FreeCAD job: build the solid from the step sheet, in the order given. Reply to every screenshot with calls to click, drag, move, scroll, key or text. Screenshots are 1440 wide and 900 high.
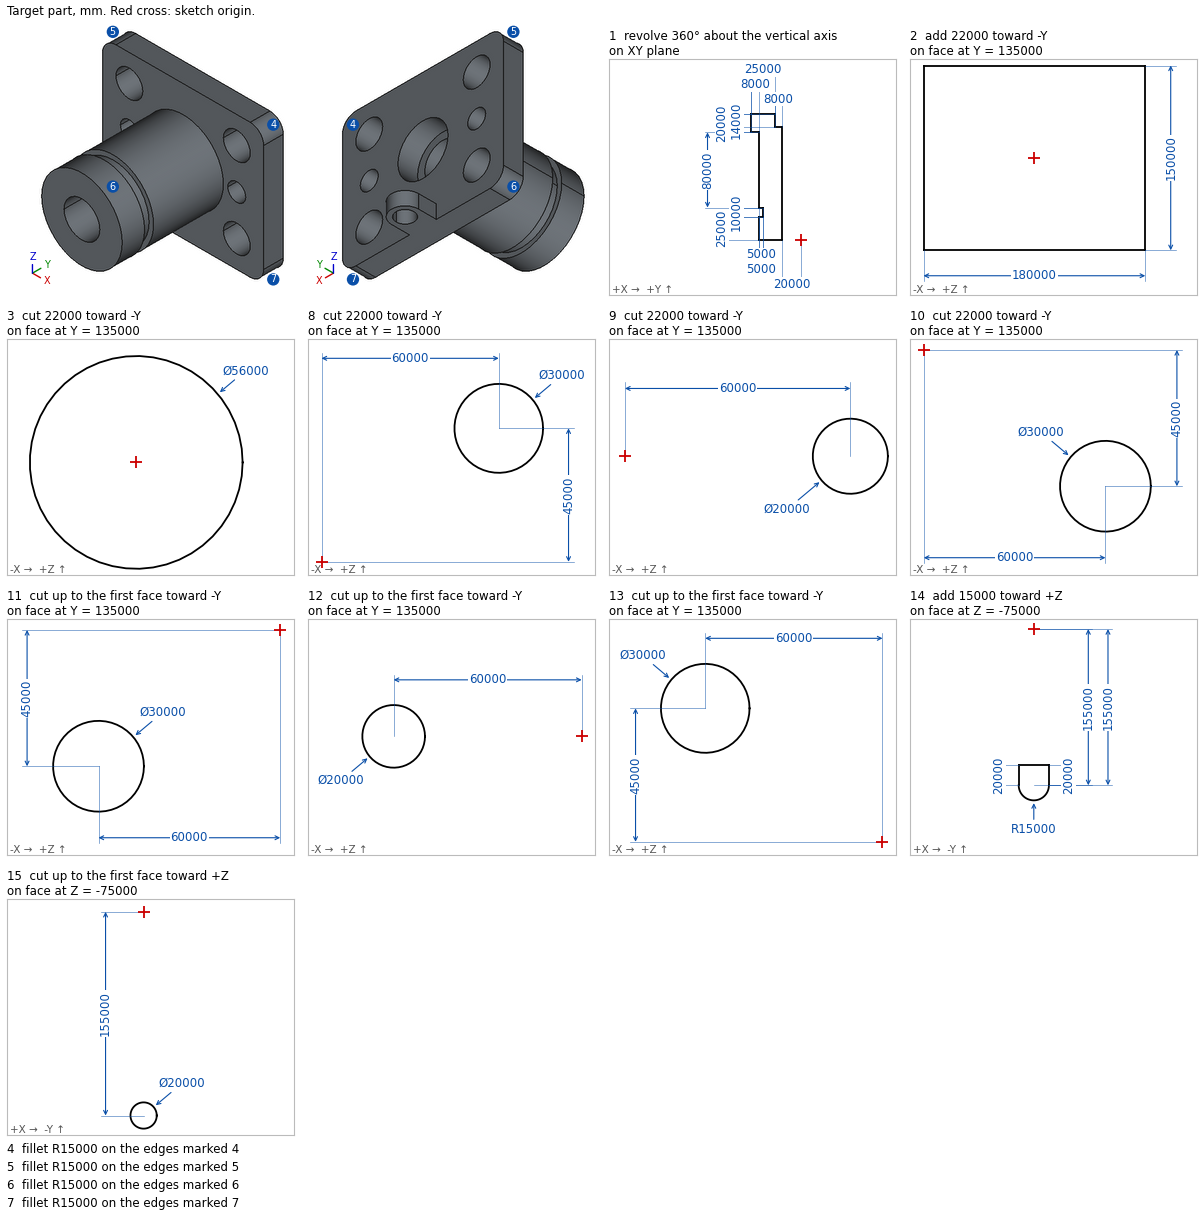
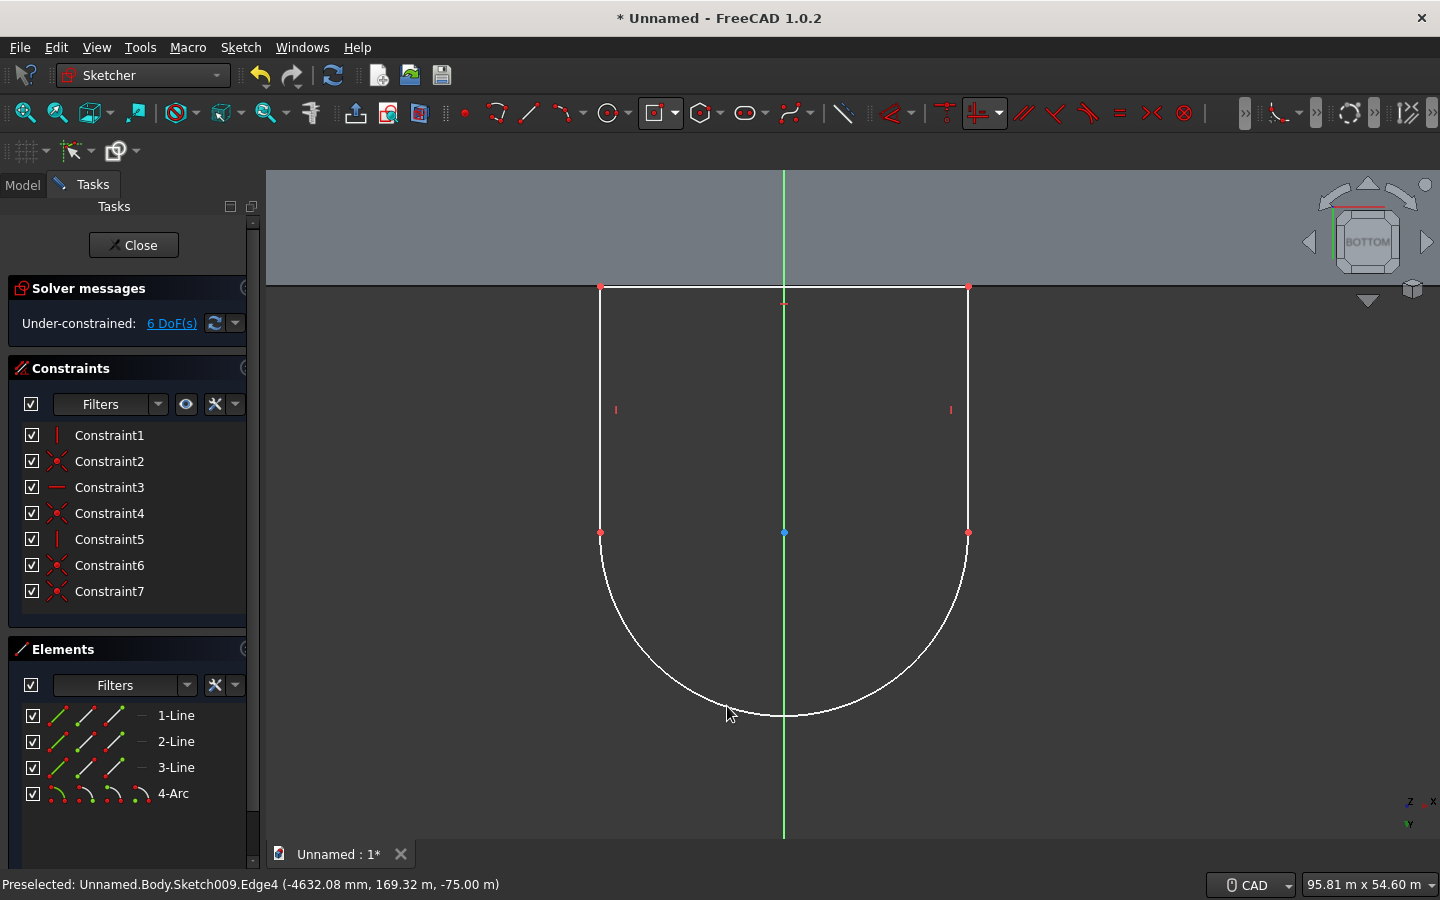
click(784, 532)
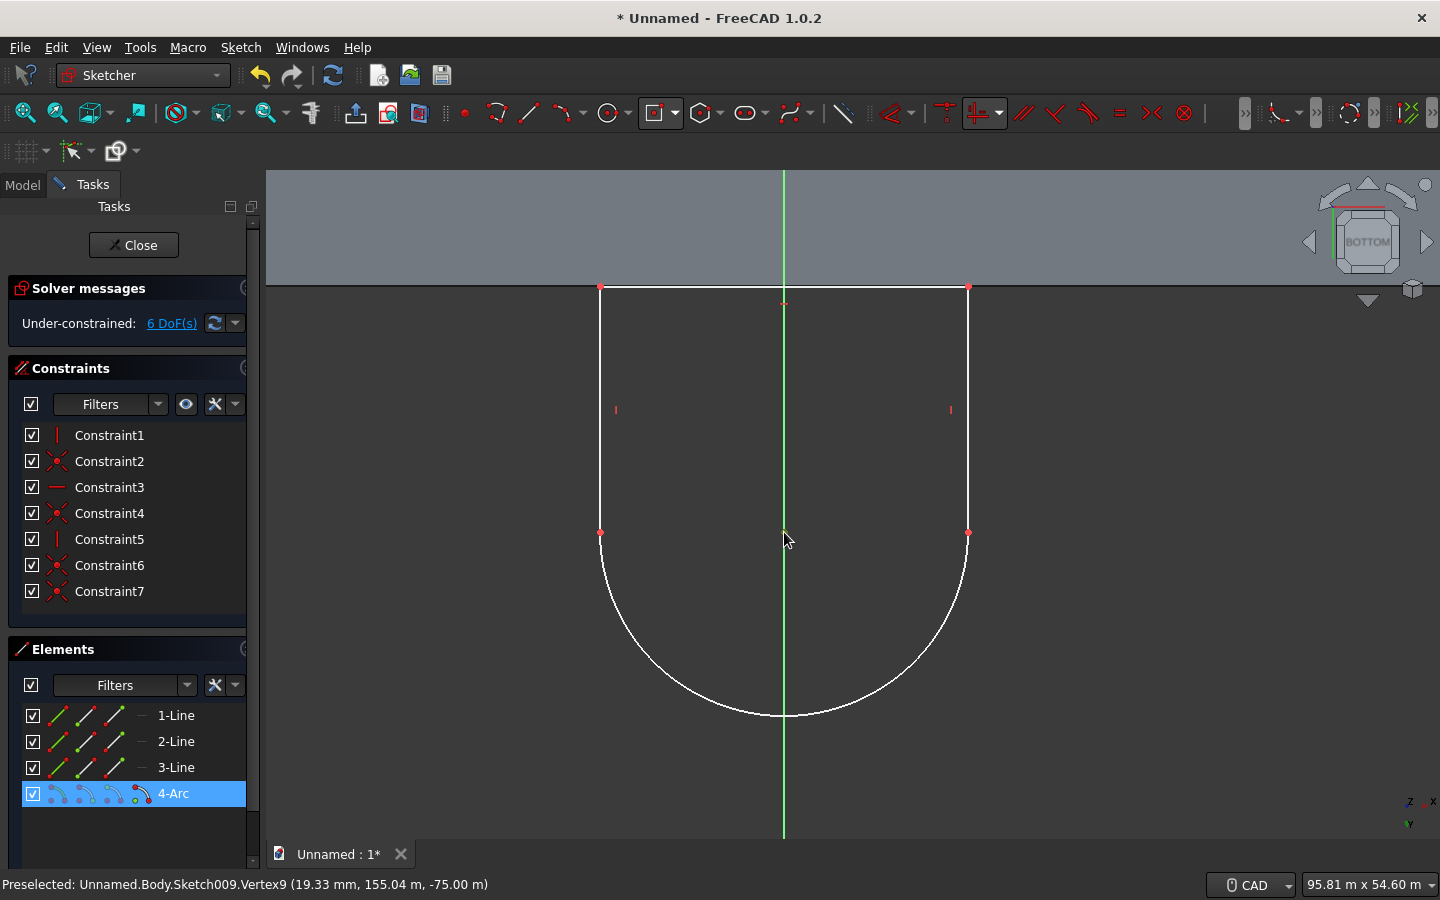
click(784, 767)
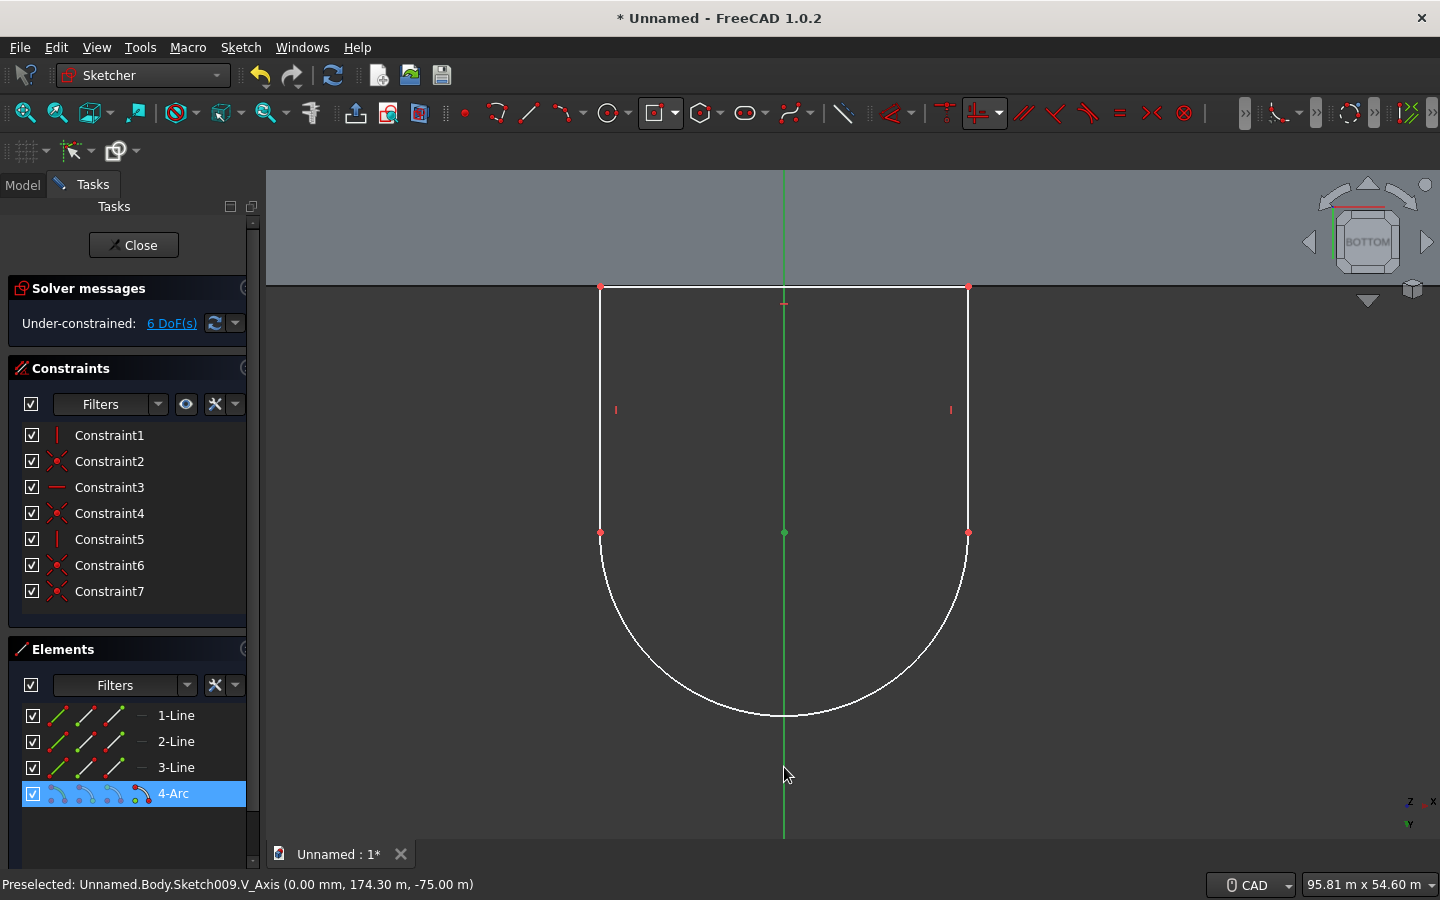
click(946, 114)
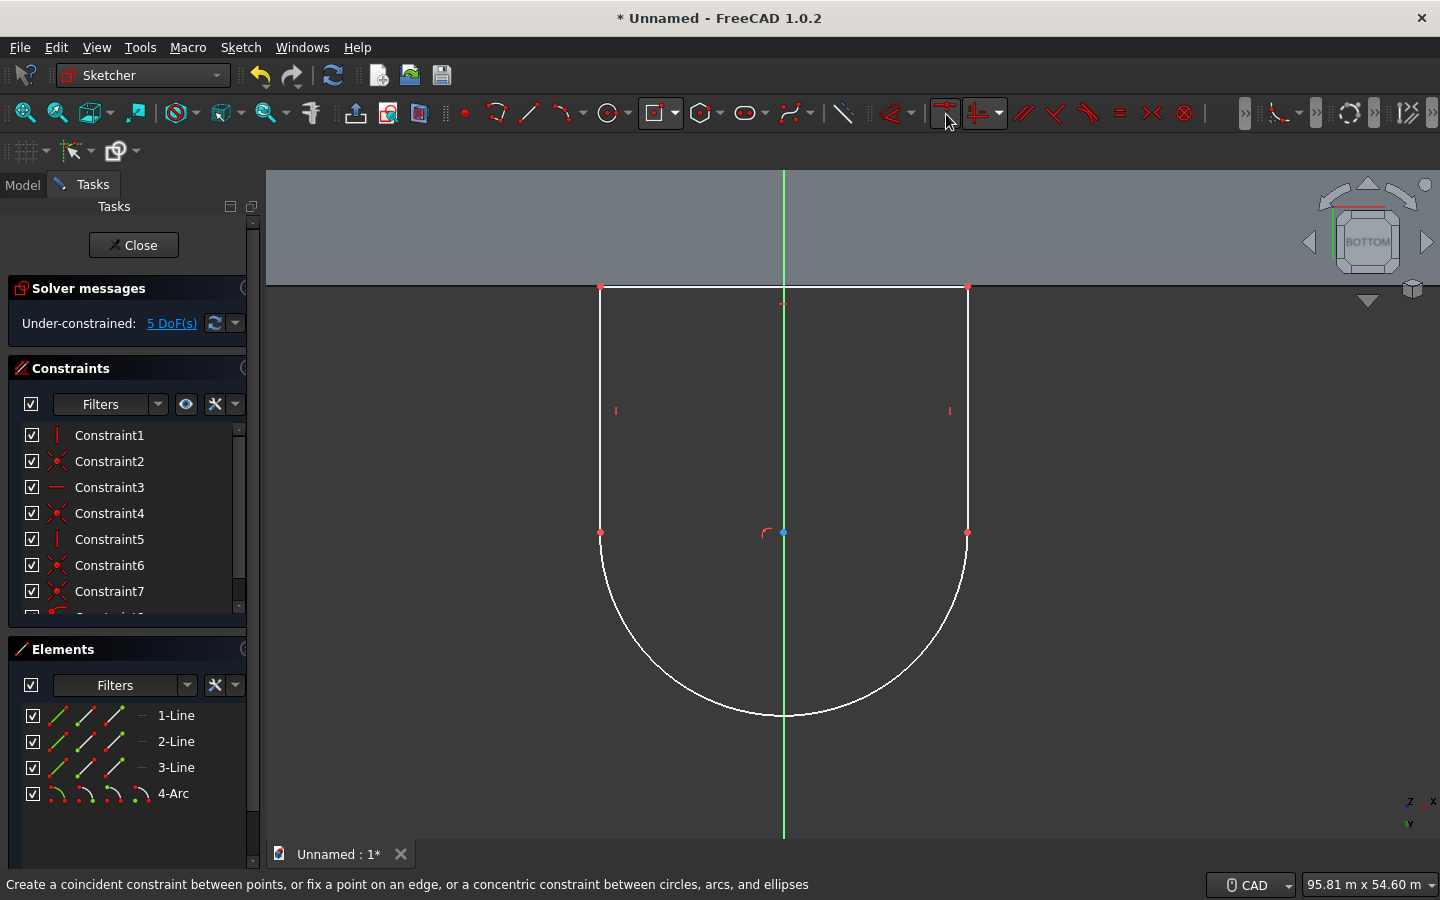
key(d)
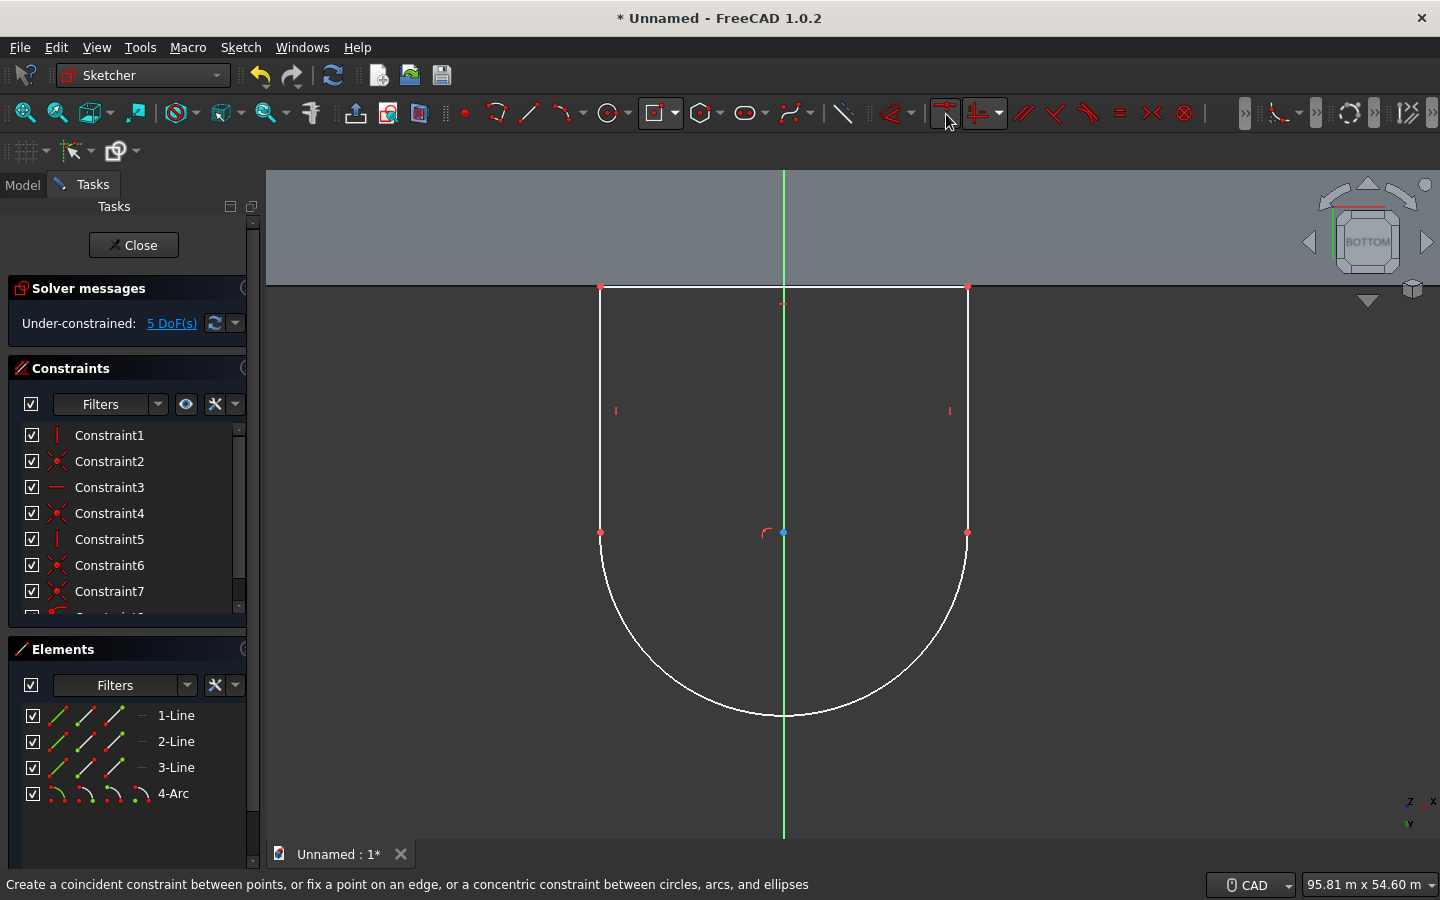
click(676, 681)
click(657, 707)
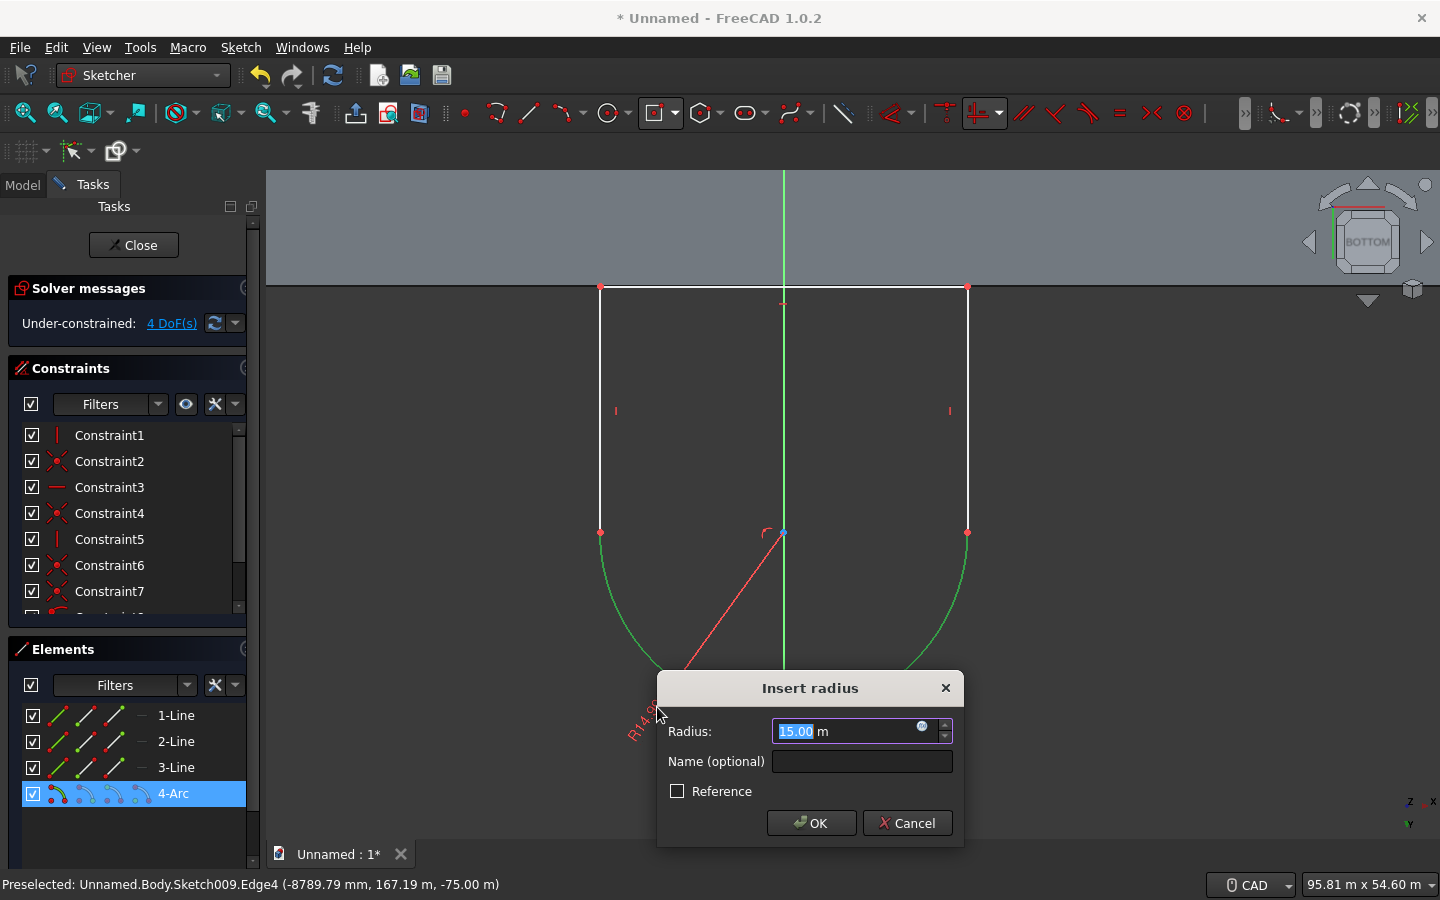
key(ctrl+a)
text(15000 mm)
key(Return)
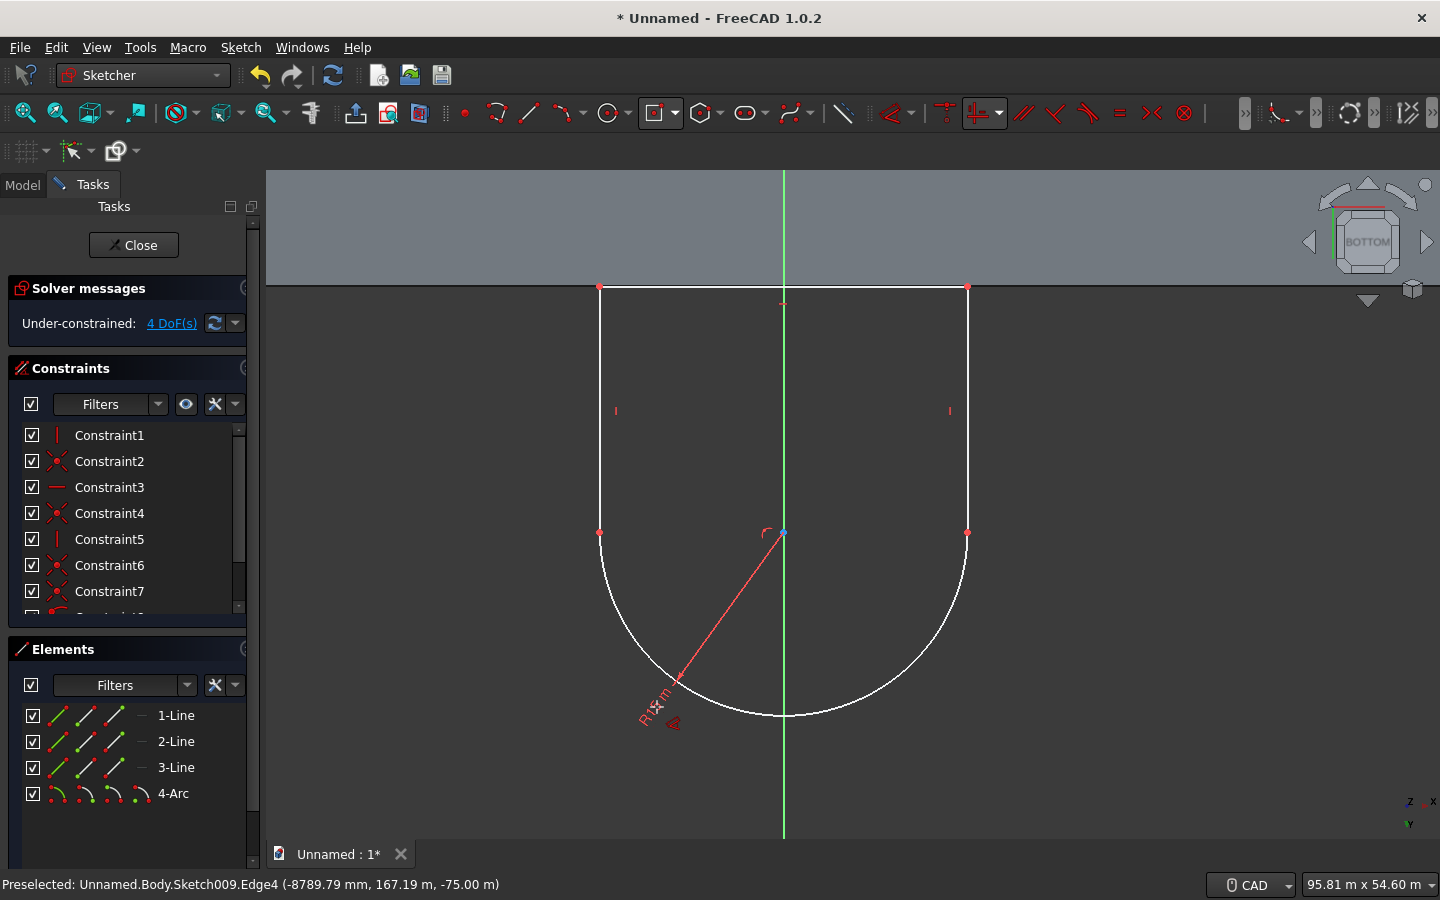
click(968, 459)
click(1002, 410)